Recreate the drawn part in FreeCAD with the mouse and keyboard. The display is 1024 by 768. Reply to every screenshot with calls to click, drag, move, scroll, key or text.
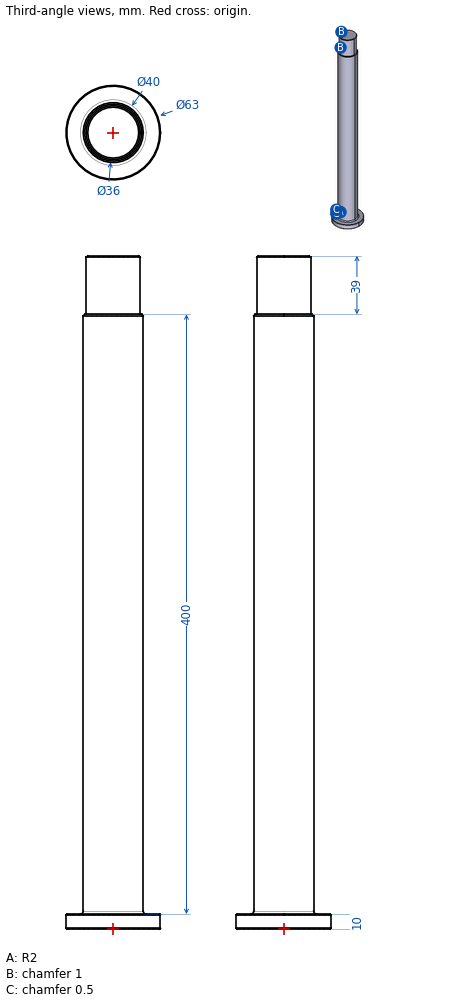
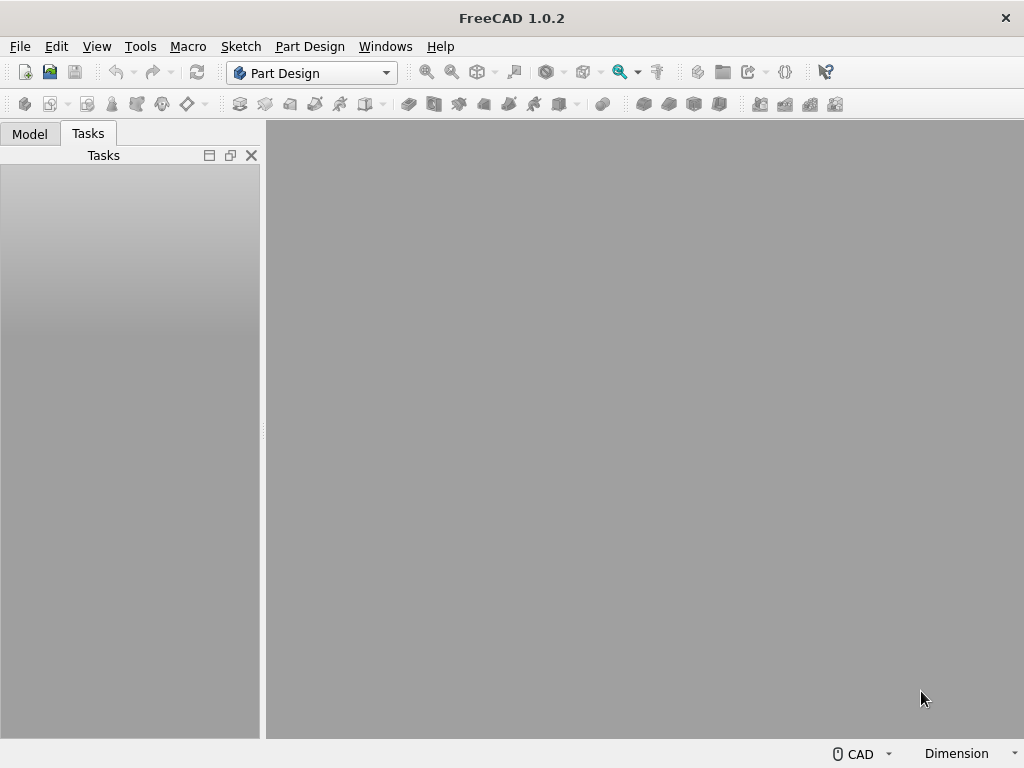
click(25, 72)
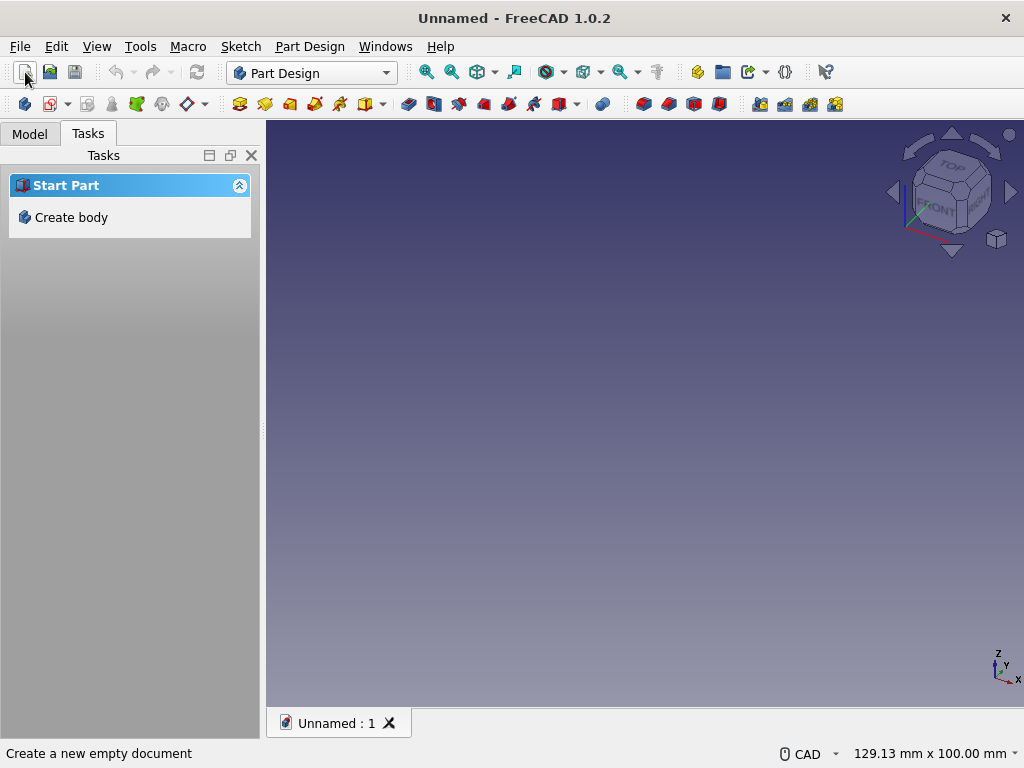
click(50, 104)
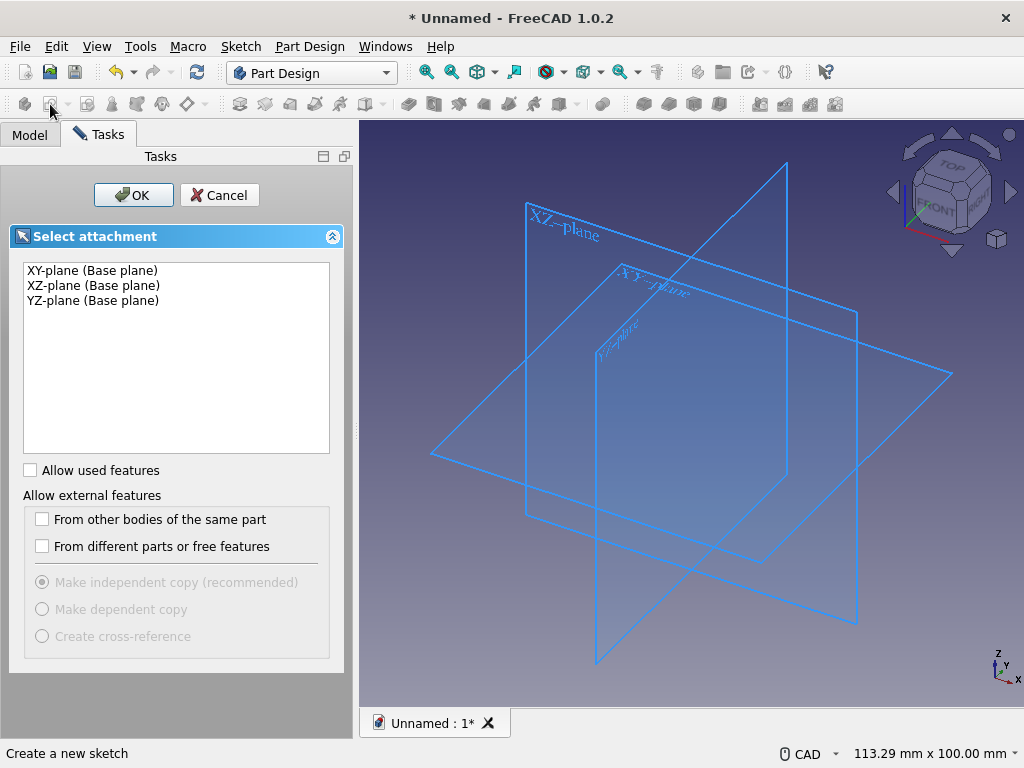
click(84, 270)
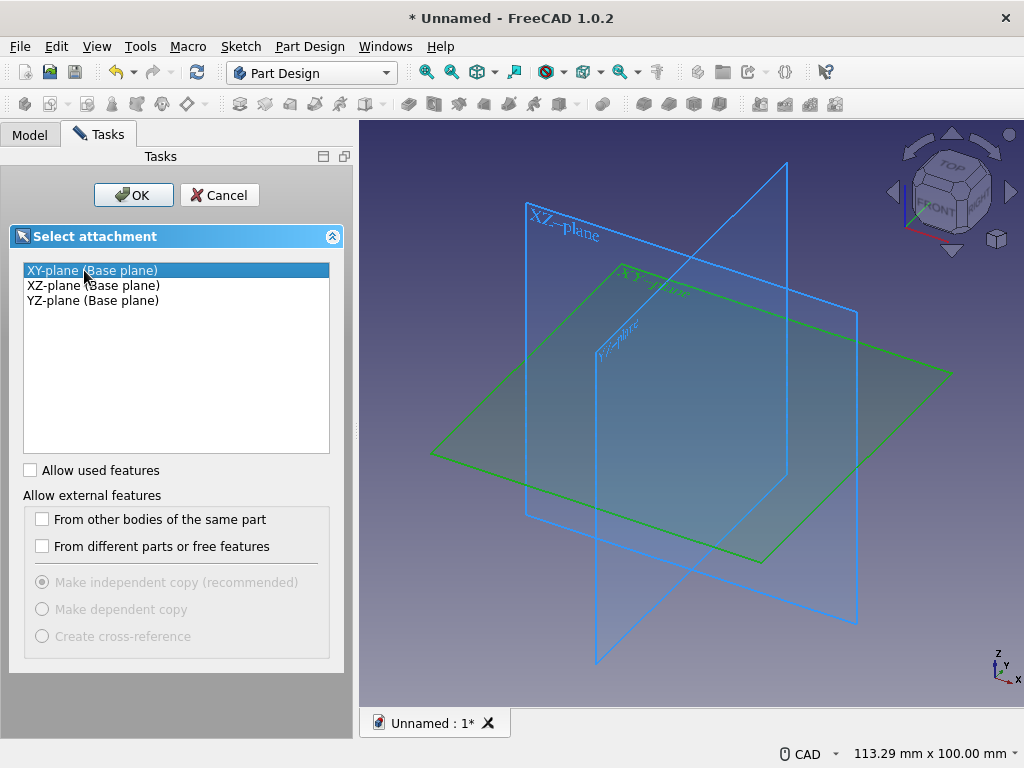
click(134, 195)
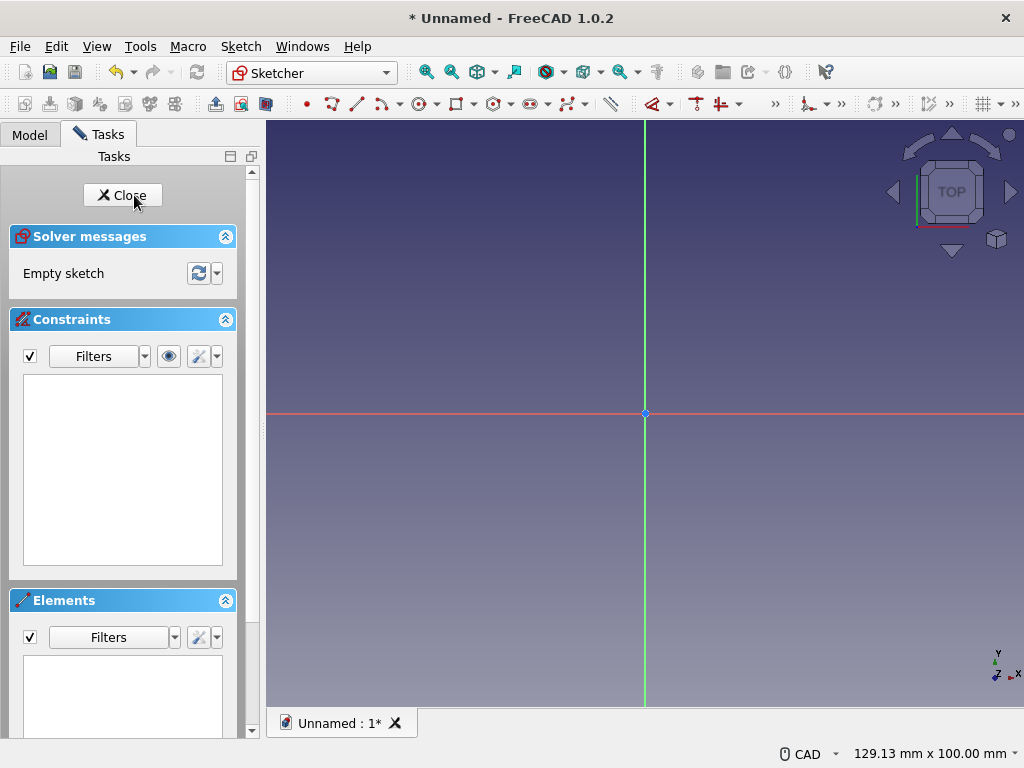
click(418, 104)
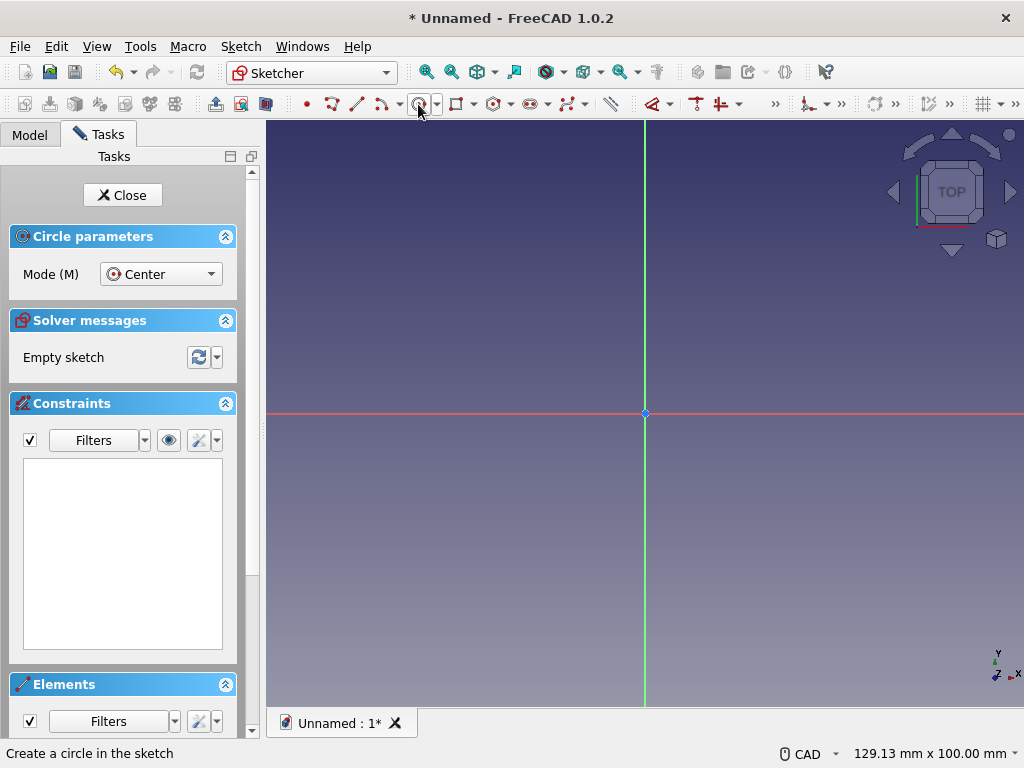
click(645, 414)
move(776, 283)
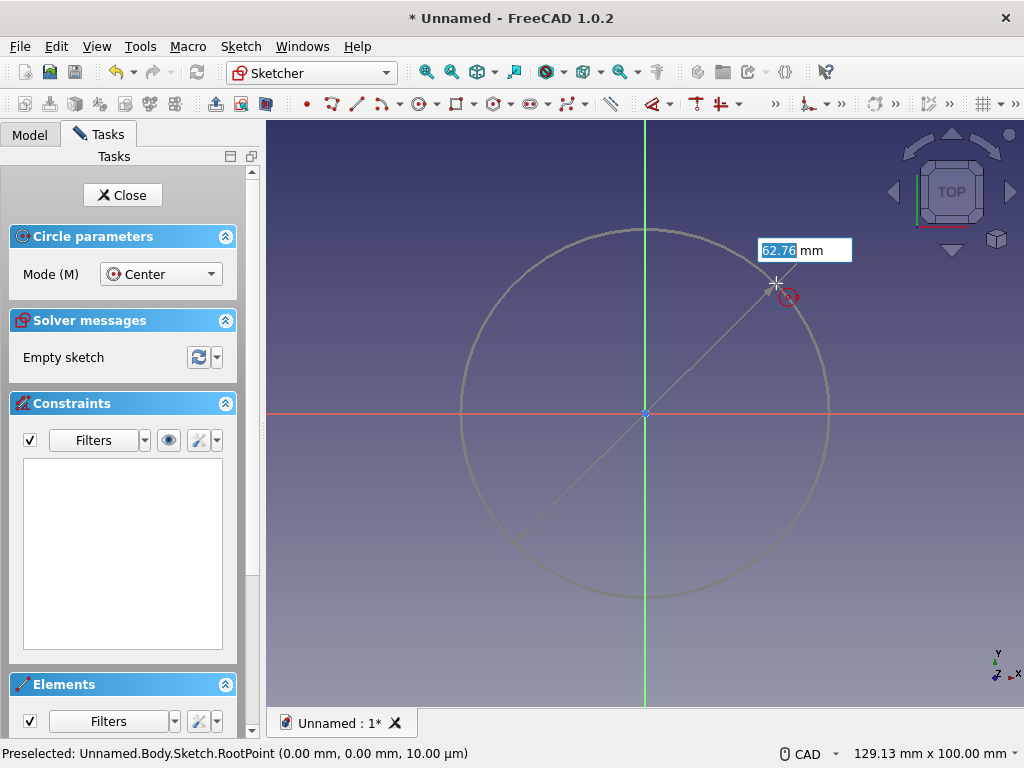
text(63)
key(Return)
key(Escape)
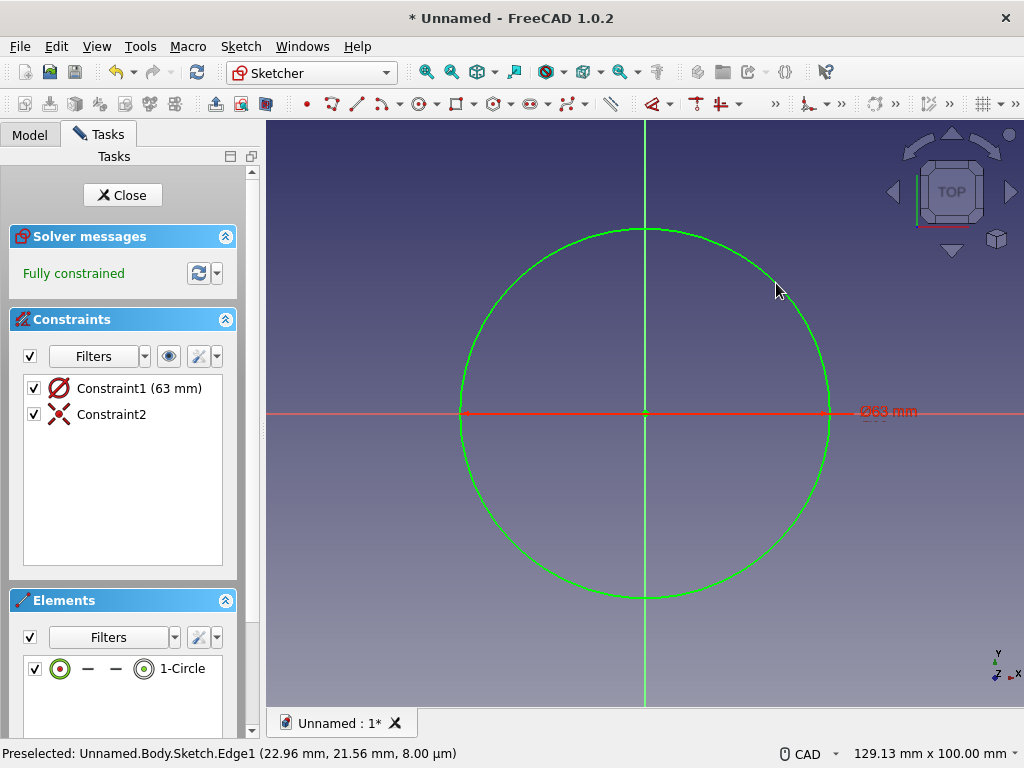
click(123, 195)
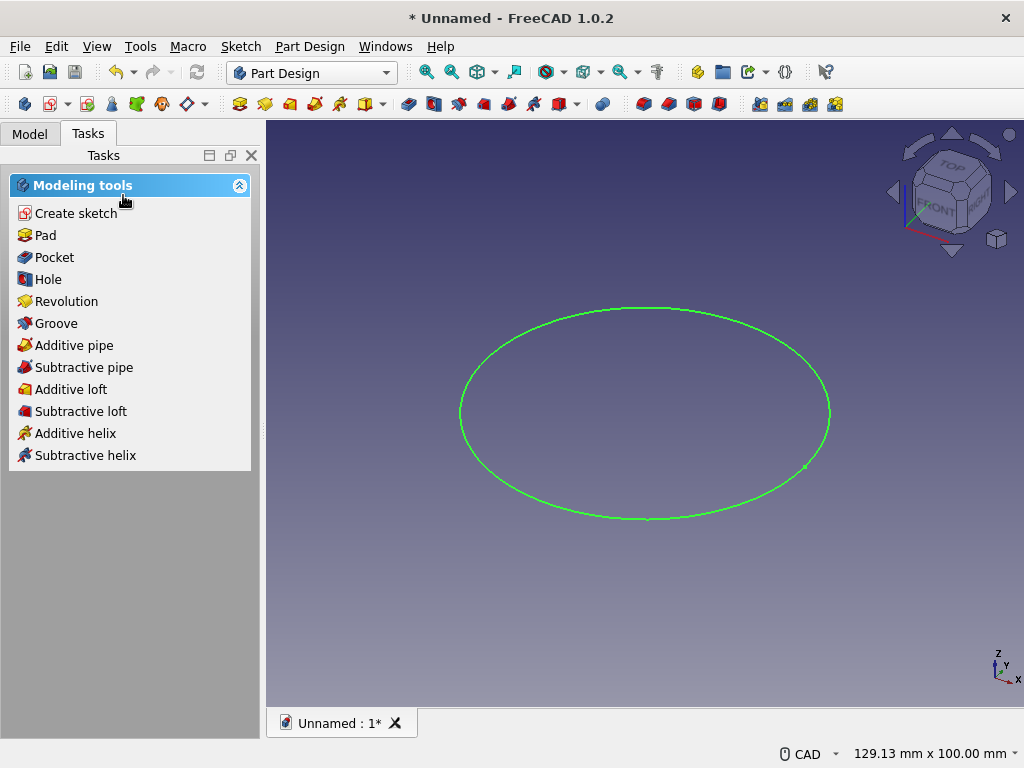
click(240, 104)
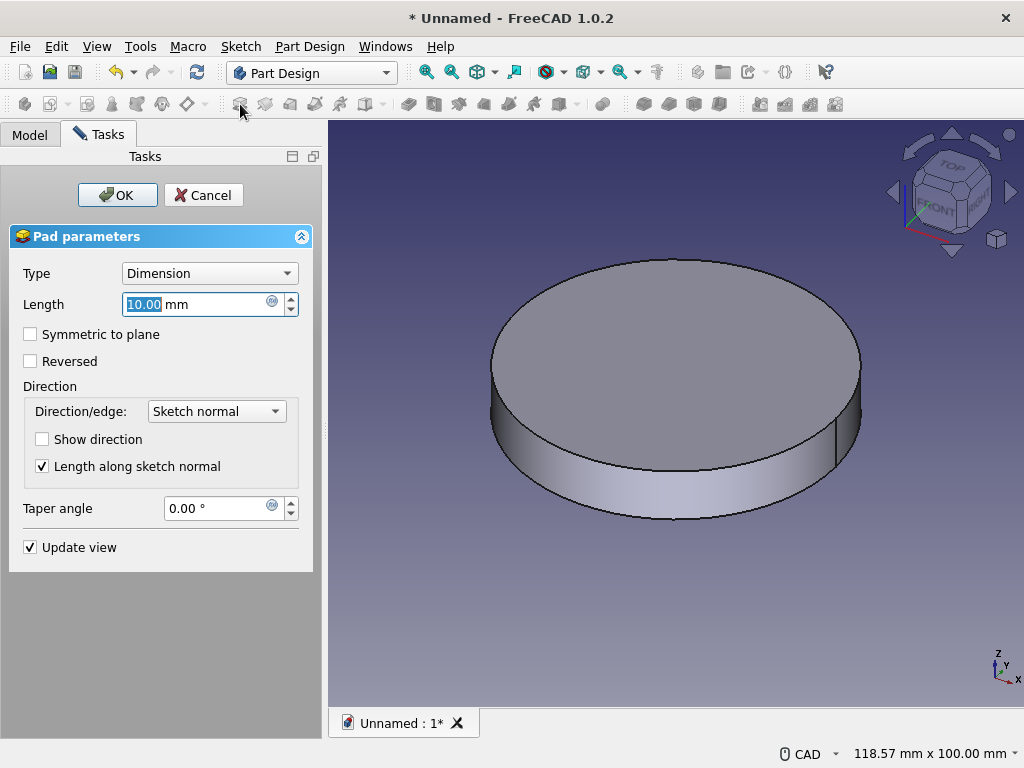
text(10)
key(Tab)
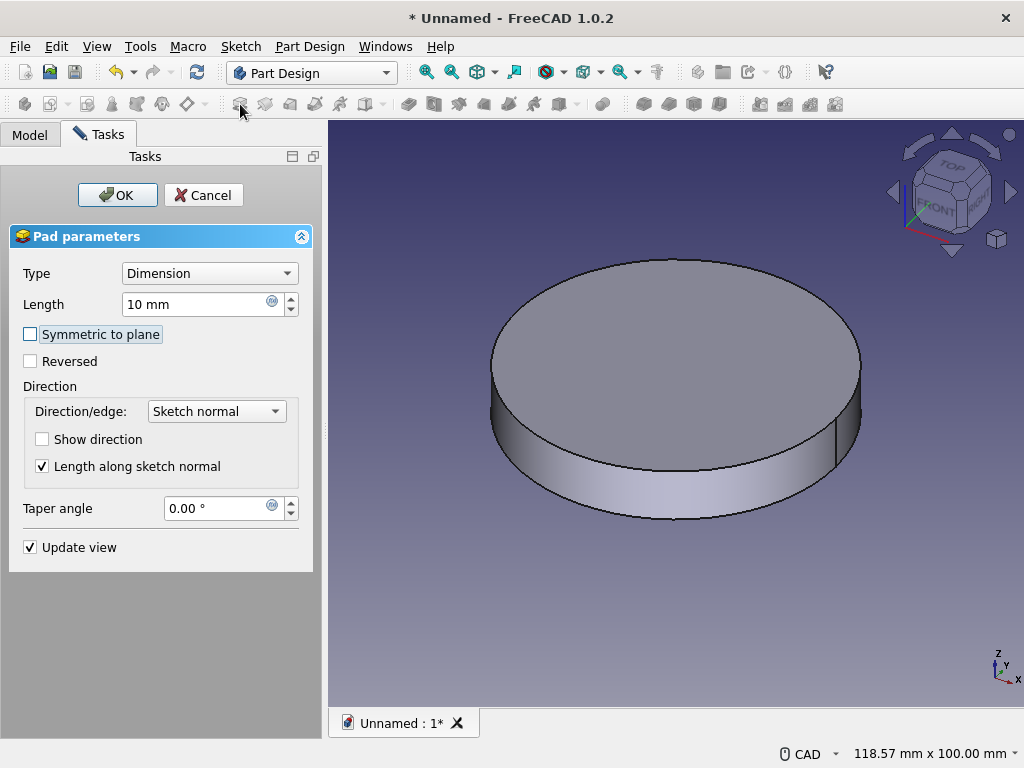
click(118, 195)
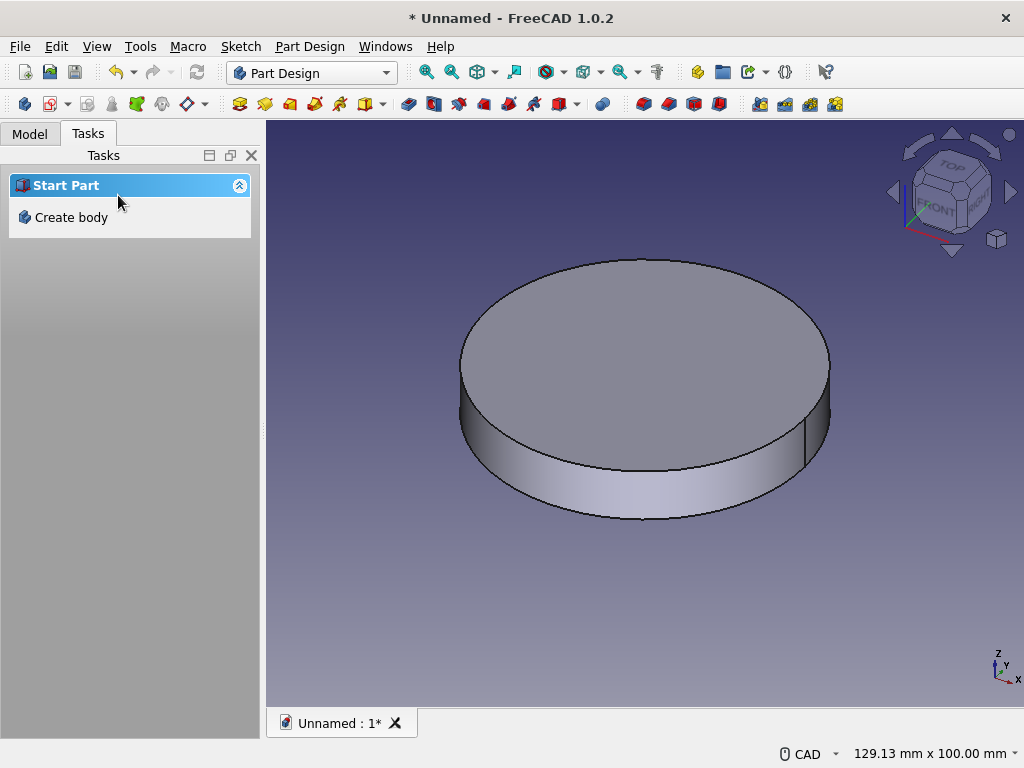
click(645, 364)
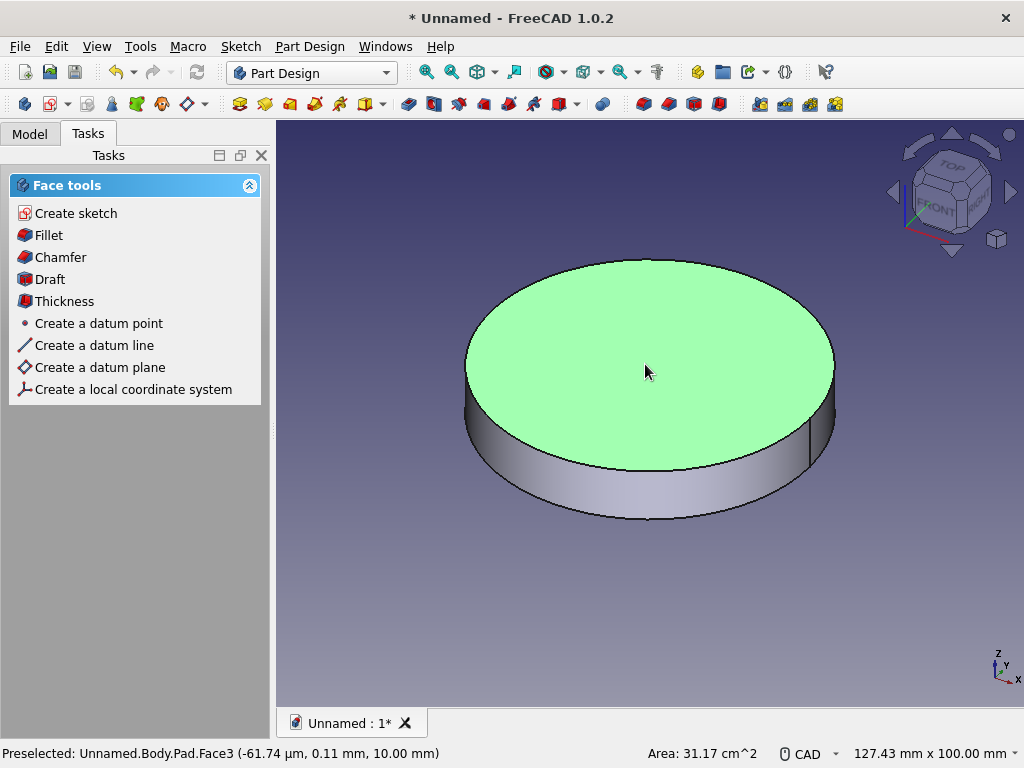
click(50, 104)